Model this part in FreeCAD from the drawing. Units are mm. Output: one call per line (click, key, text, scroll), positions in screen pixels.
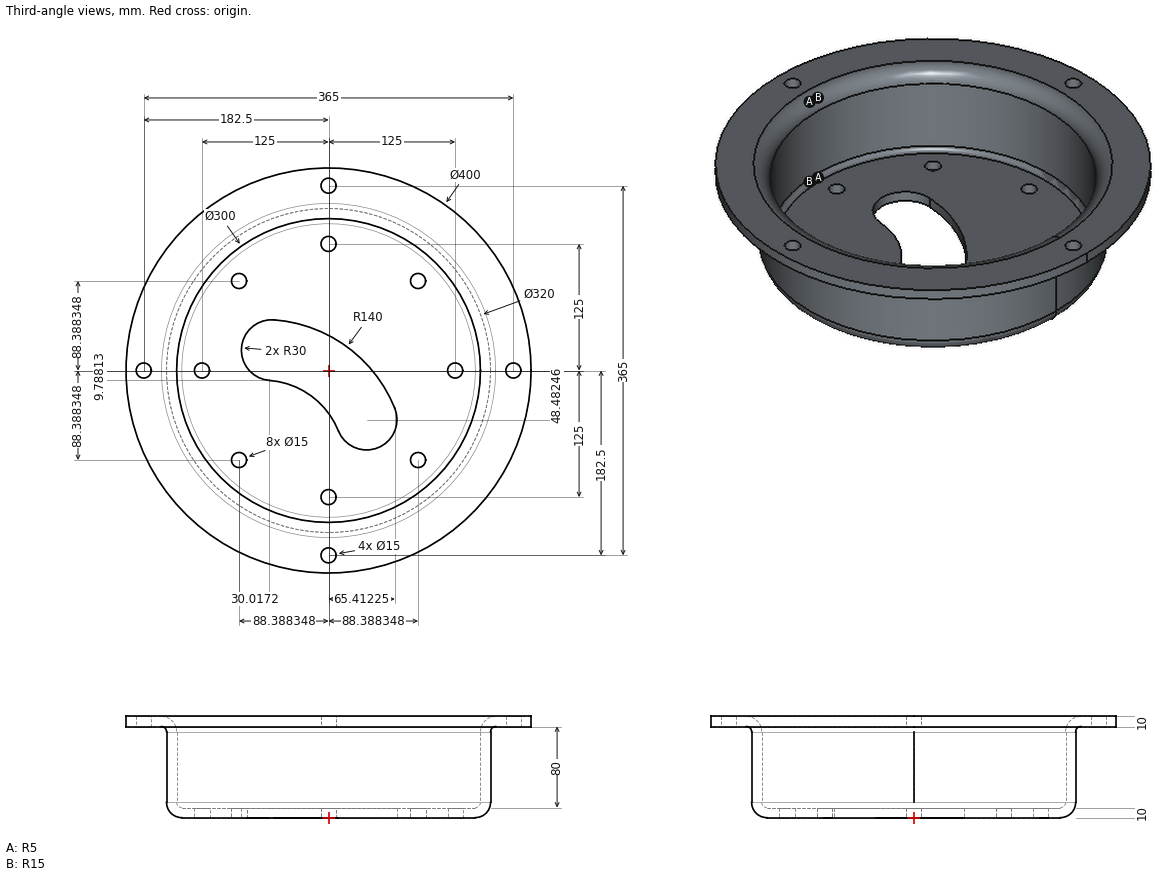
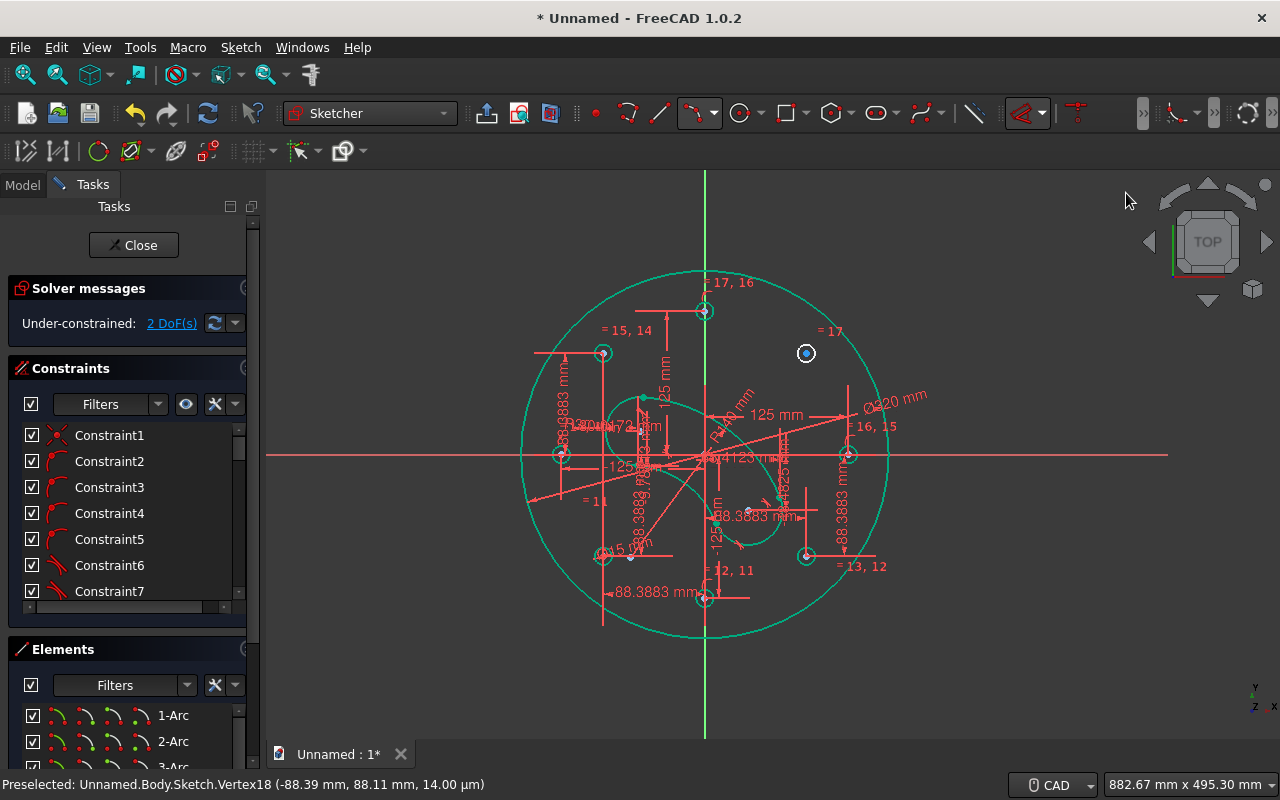
click(806, 353)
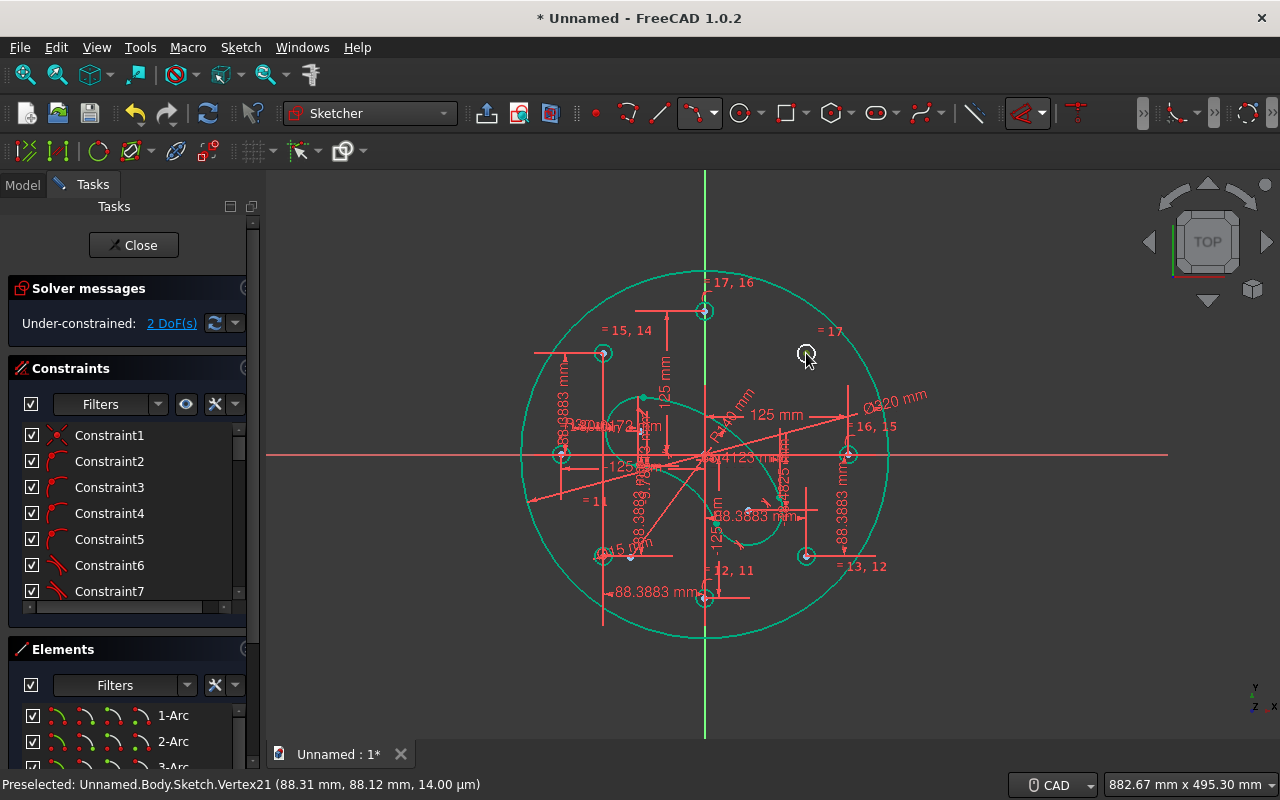
click(1044, 114)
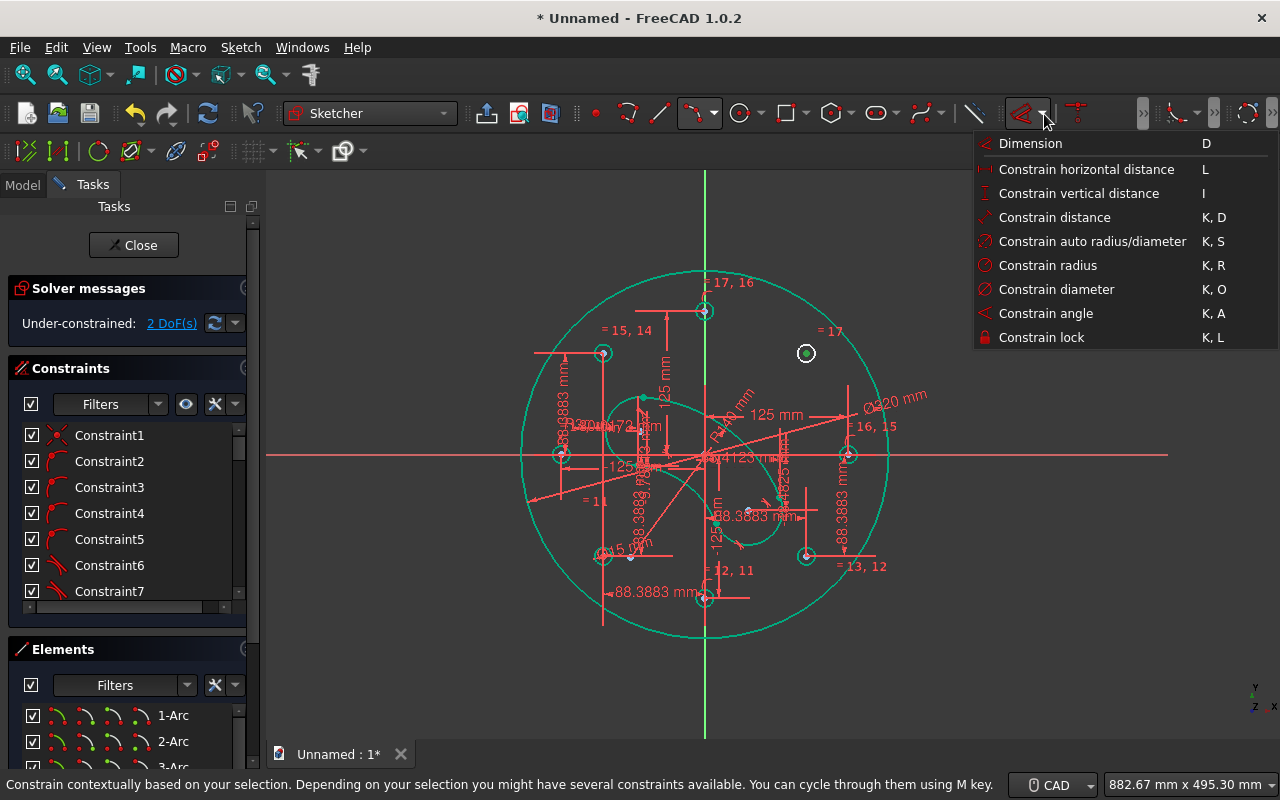
click(1126, 169)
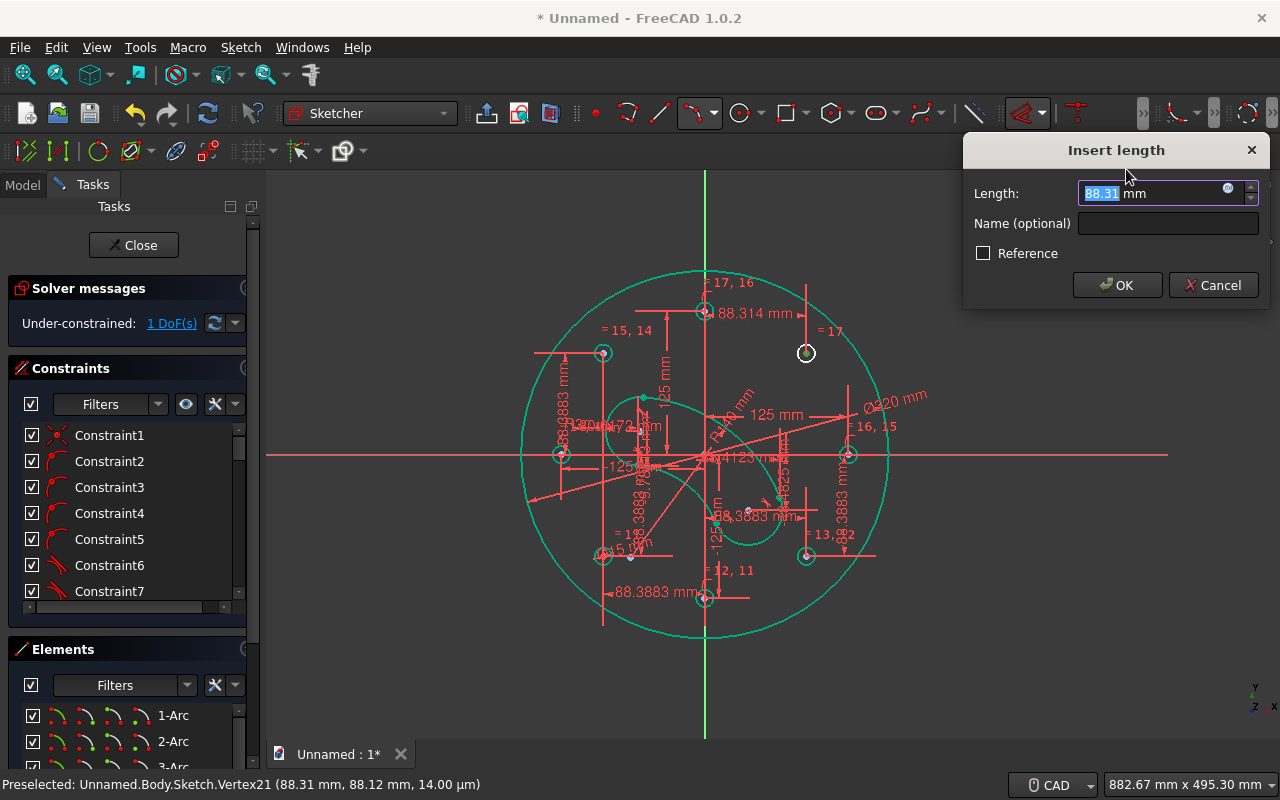
text(88.388348)
key(Return)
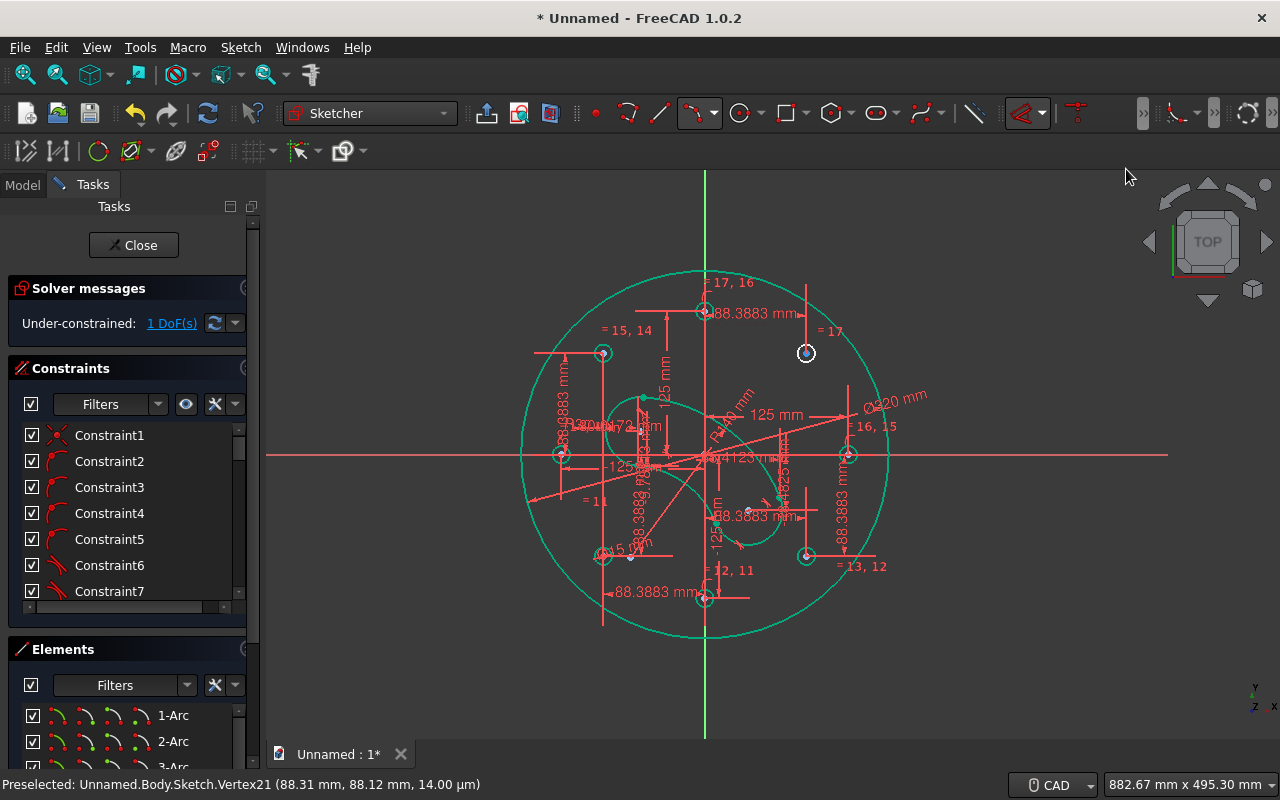
click(806, 353)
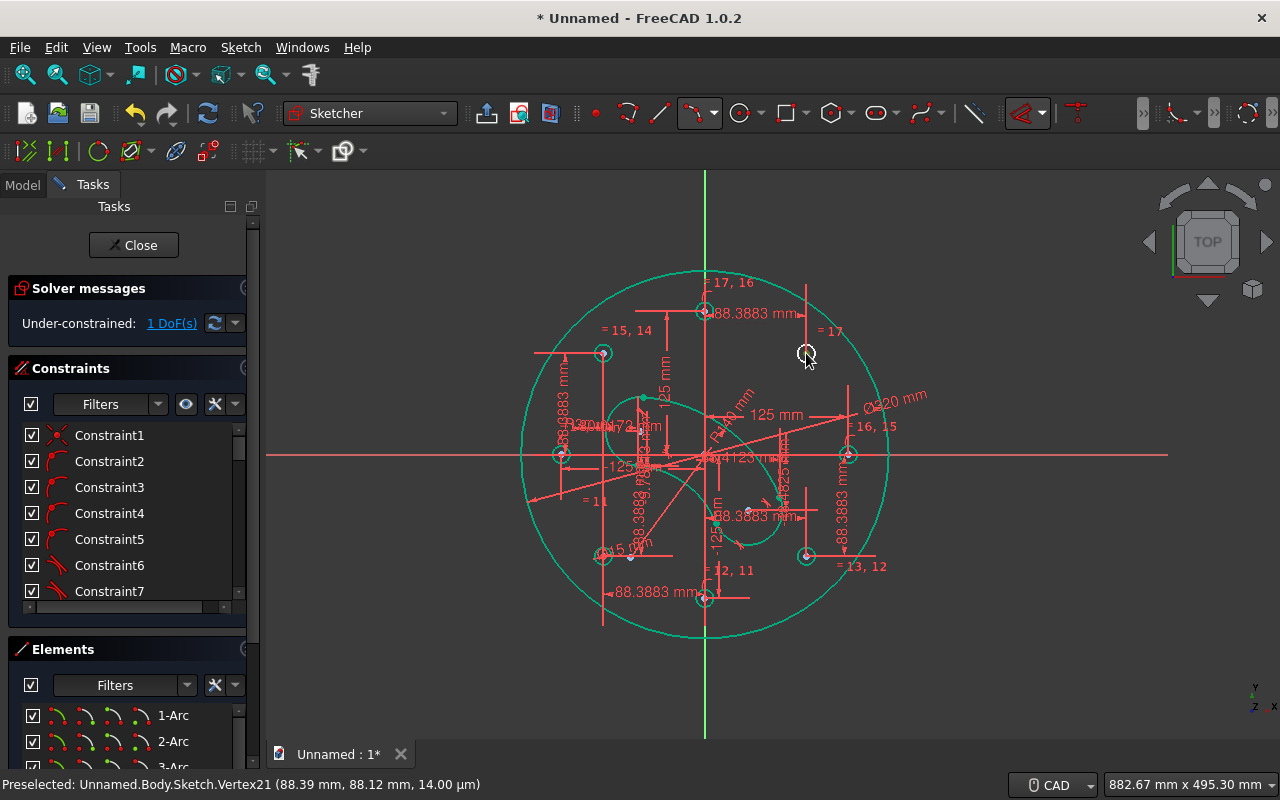
click(1044, 114)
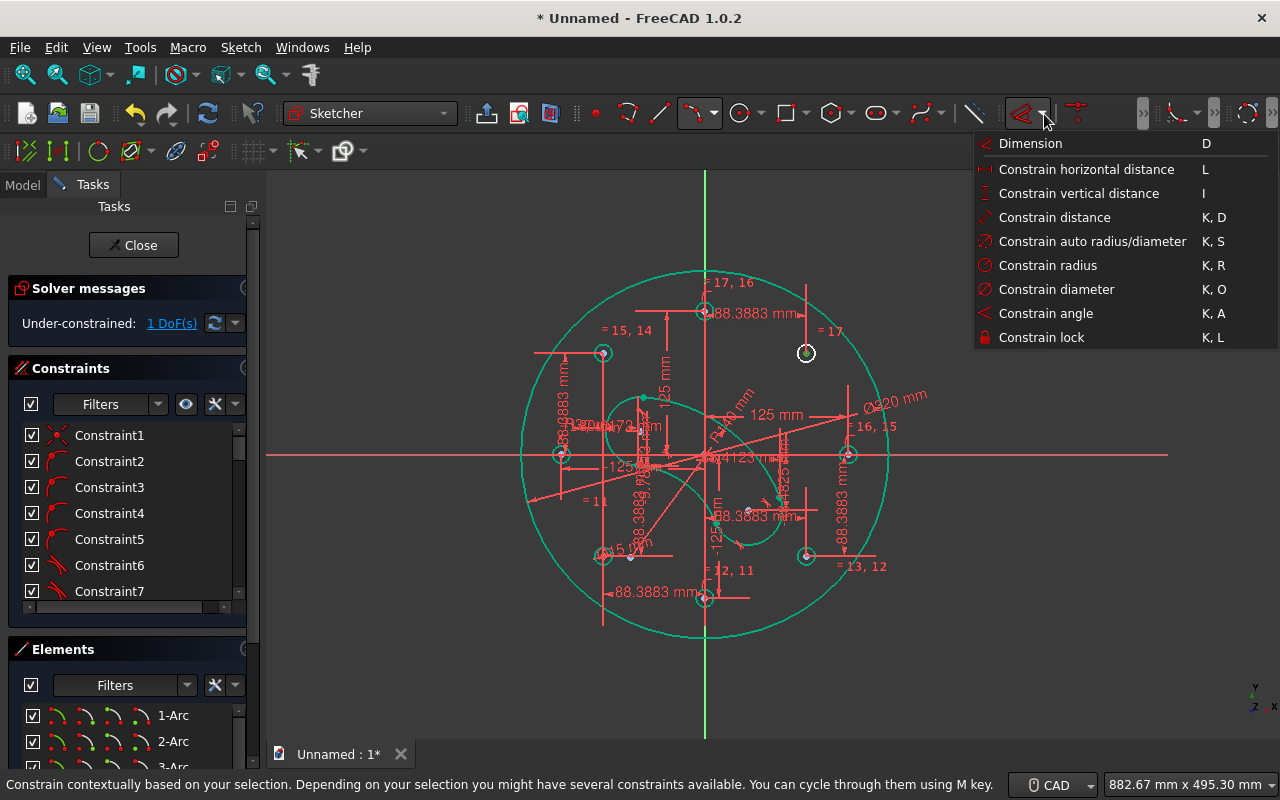
click(1126, 193)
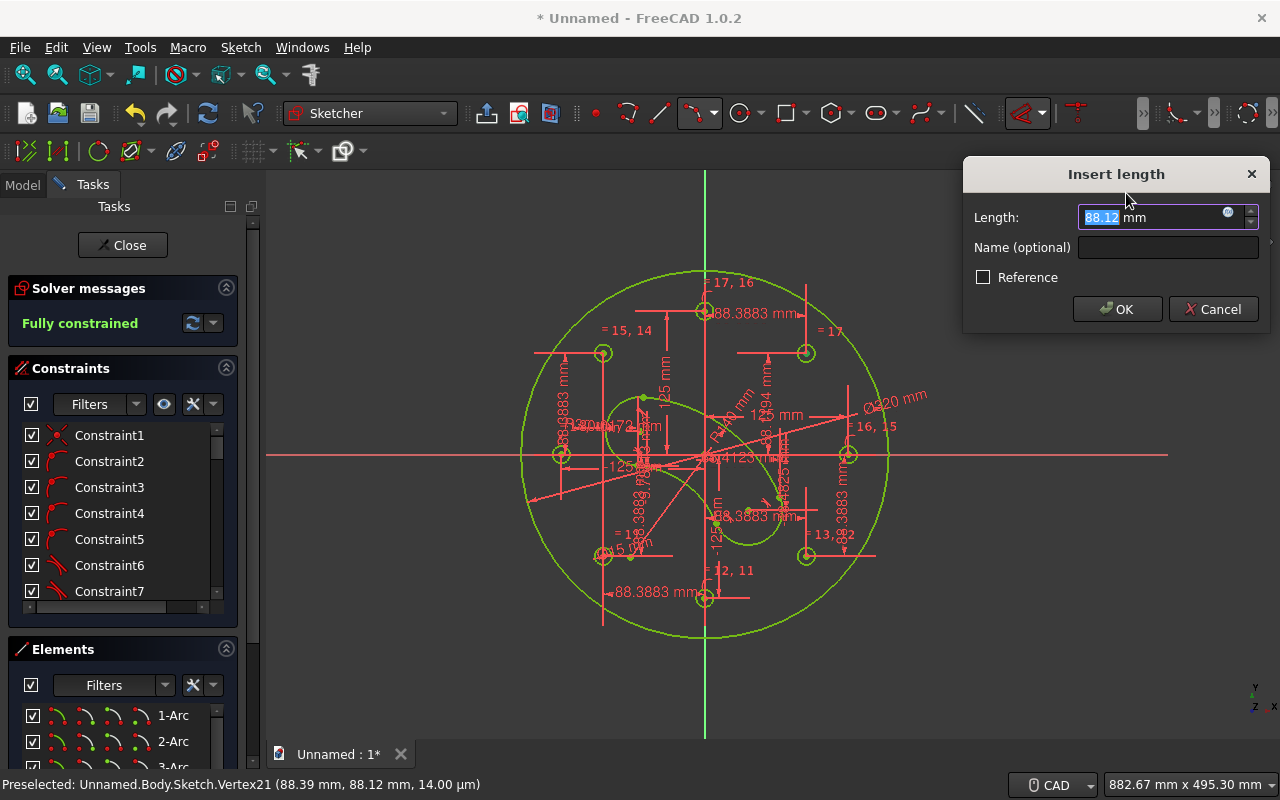
text(88.388348)
key(Return)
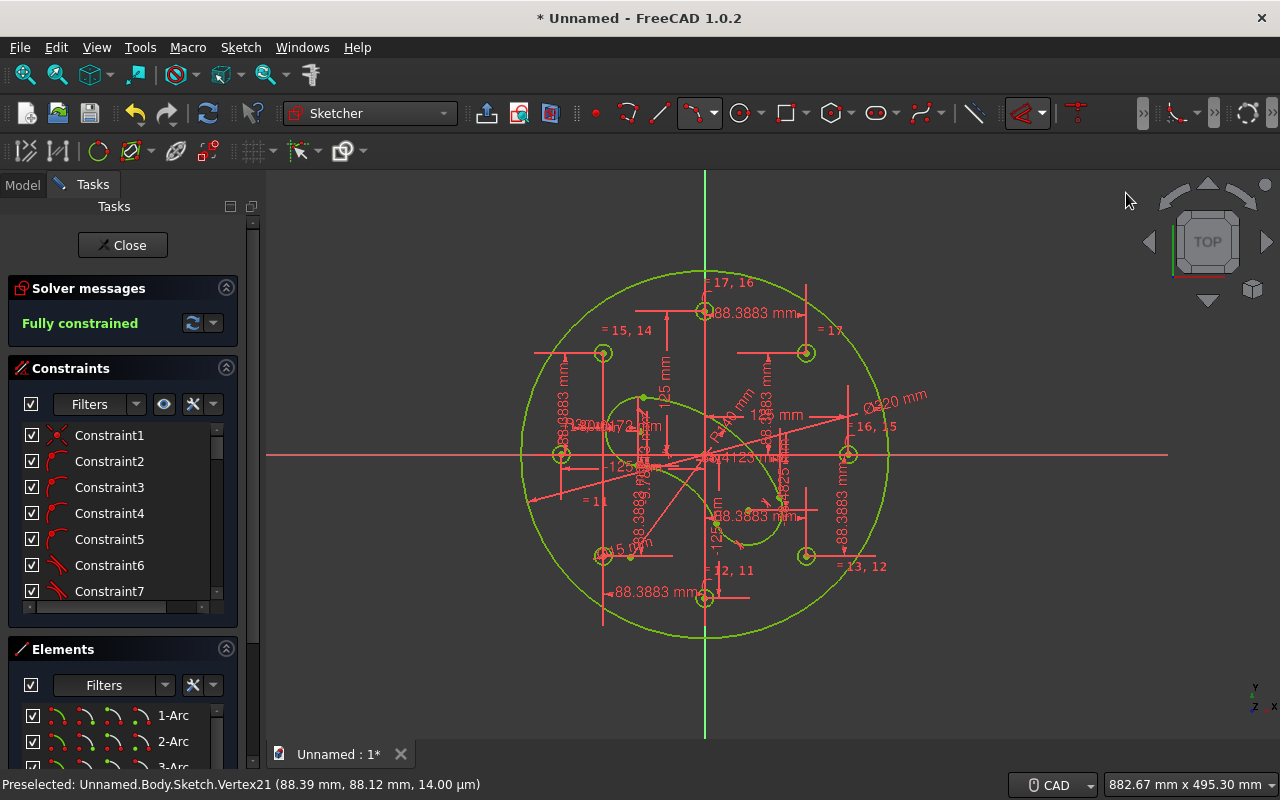
click(123, 245)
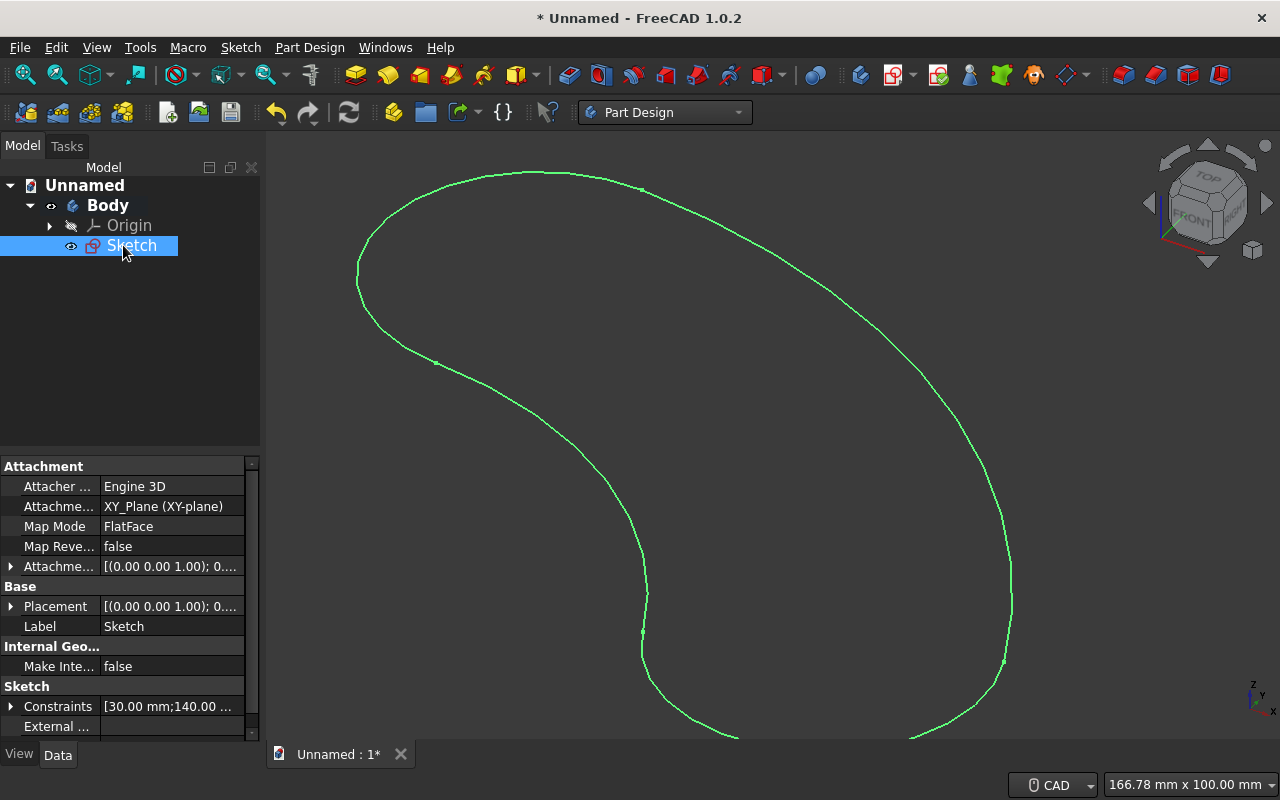
click(356, 76)